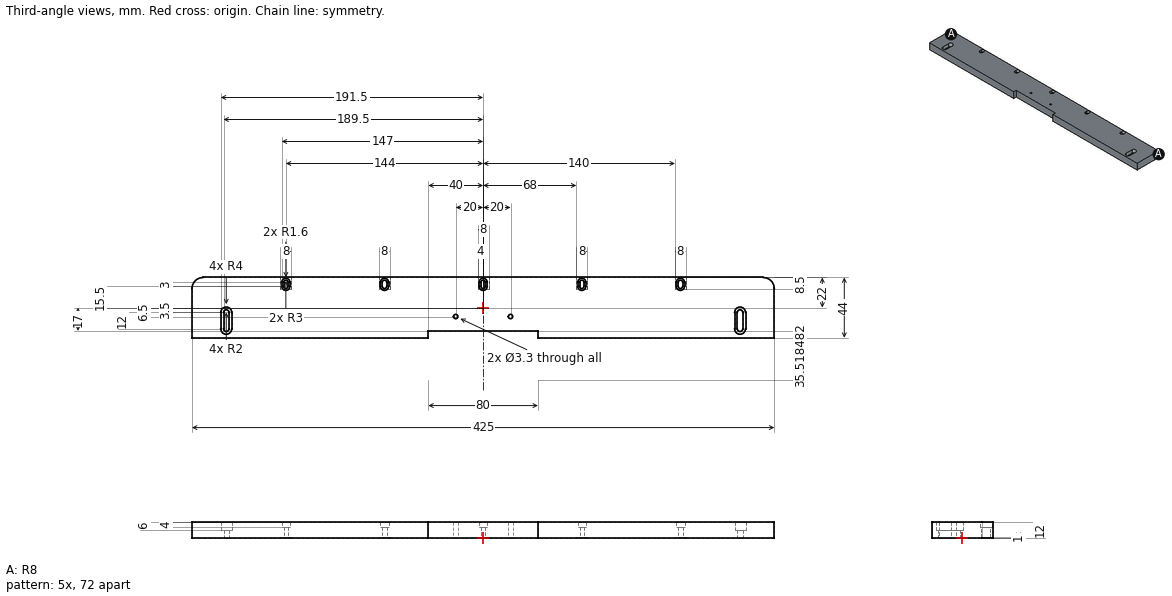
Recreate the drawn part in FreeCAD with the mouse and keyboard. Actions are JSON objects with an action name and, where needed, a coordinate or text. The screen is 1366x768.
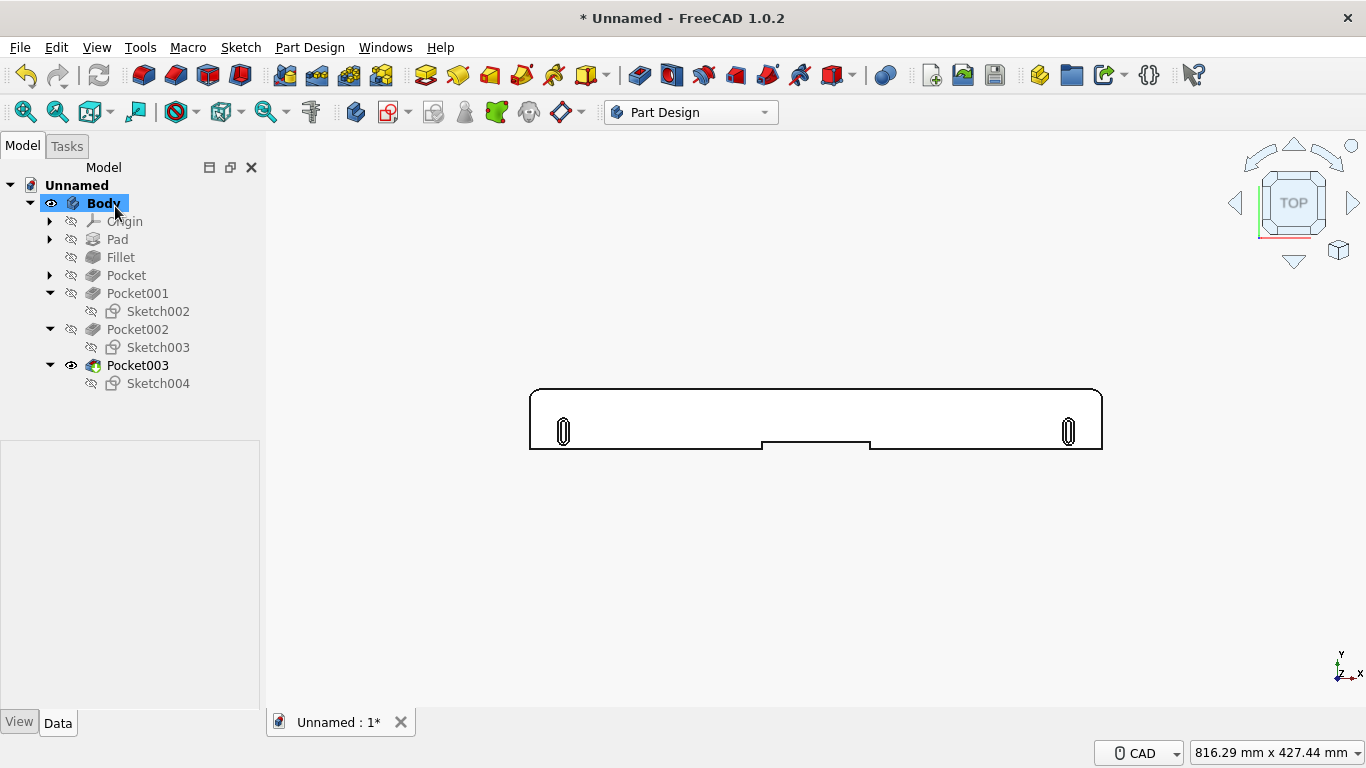
{"action": "left_click", "coordinate": [980, 418]}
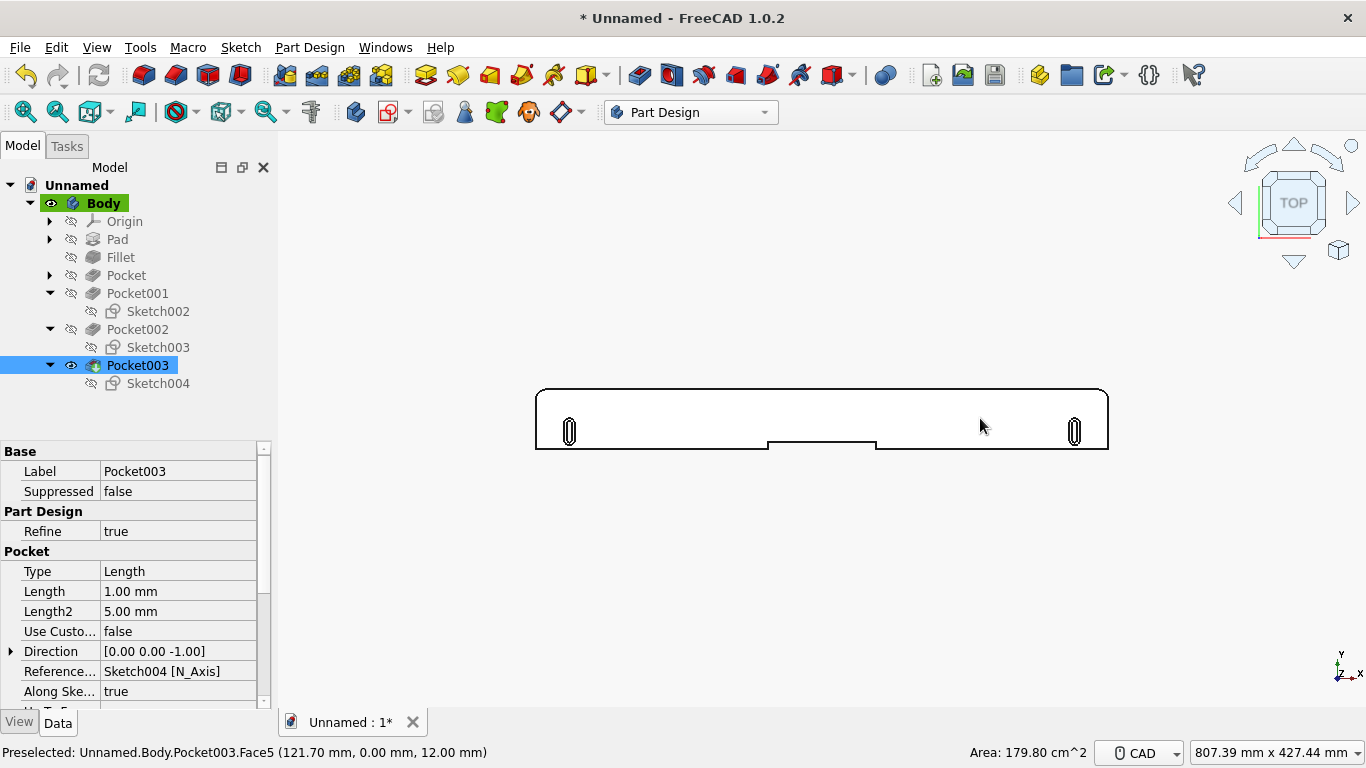
{"action": "left_click", "coordinate": [388, 112]}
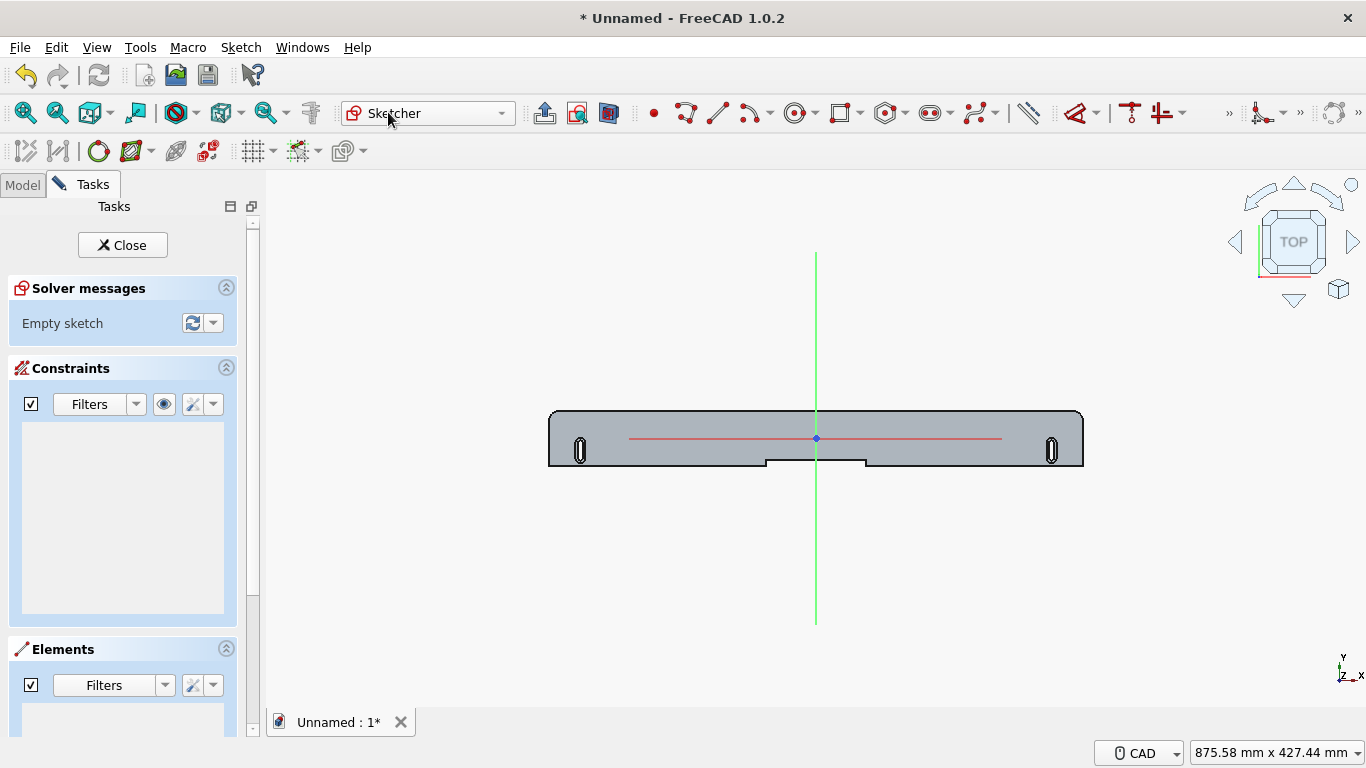
{"action": "scroll", "coordinate": [629, 416], "scroll_direction": "up", "scroll_amount": 15}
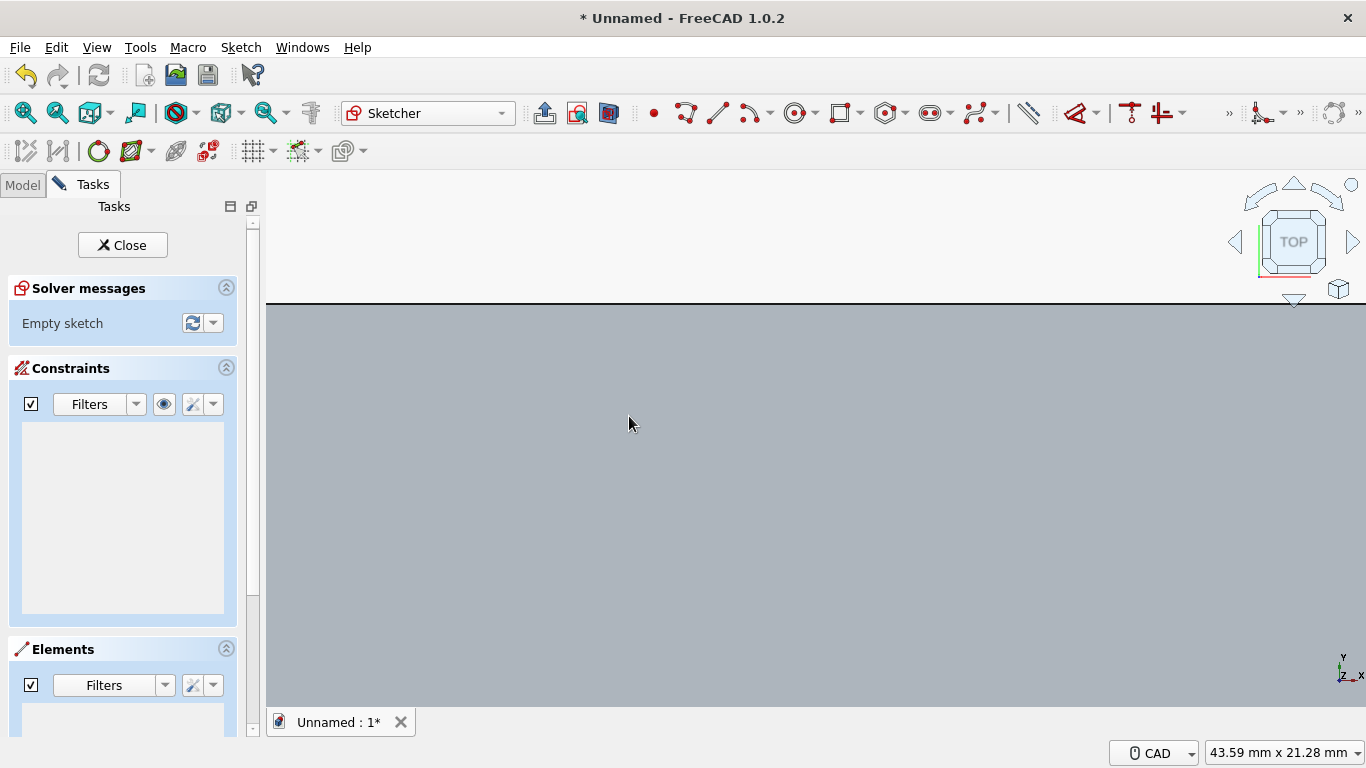
{"action": "scroll", "coordinate": [740, 413], "scroll_direction": "up", "scroll_amount": 2}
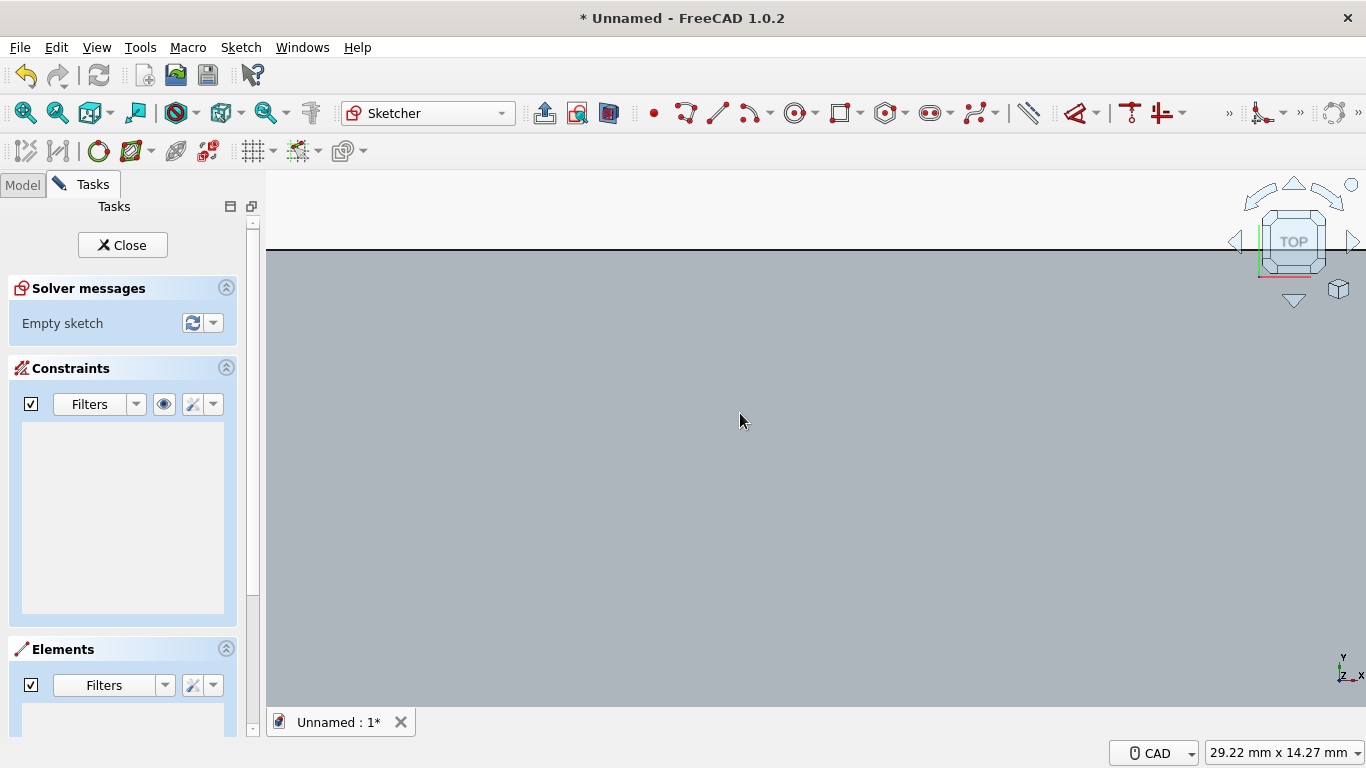
{"action": "left_click", "coordinate": [930, 114]}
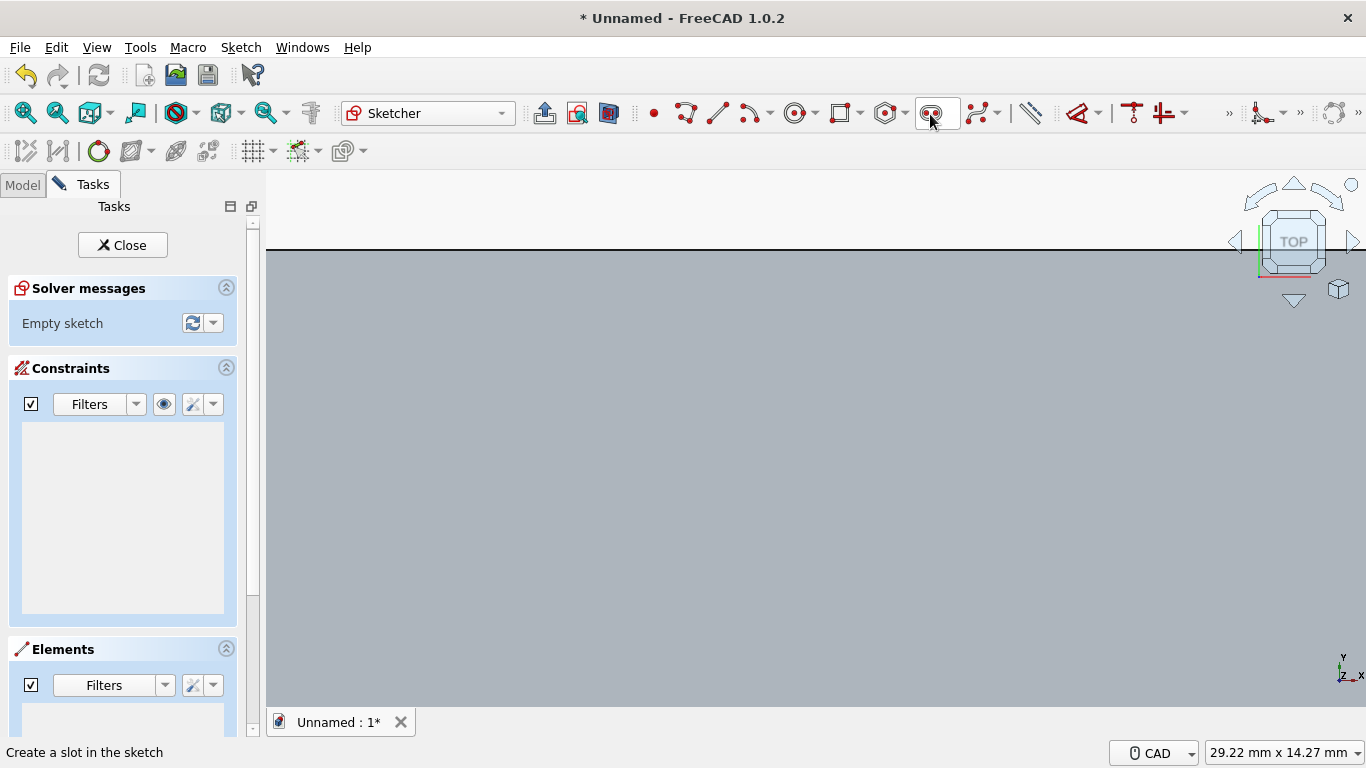
{"action": "left_click", "coordinate": [747, 495]}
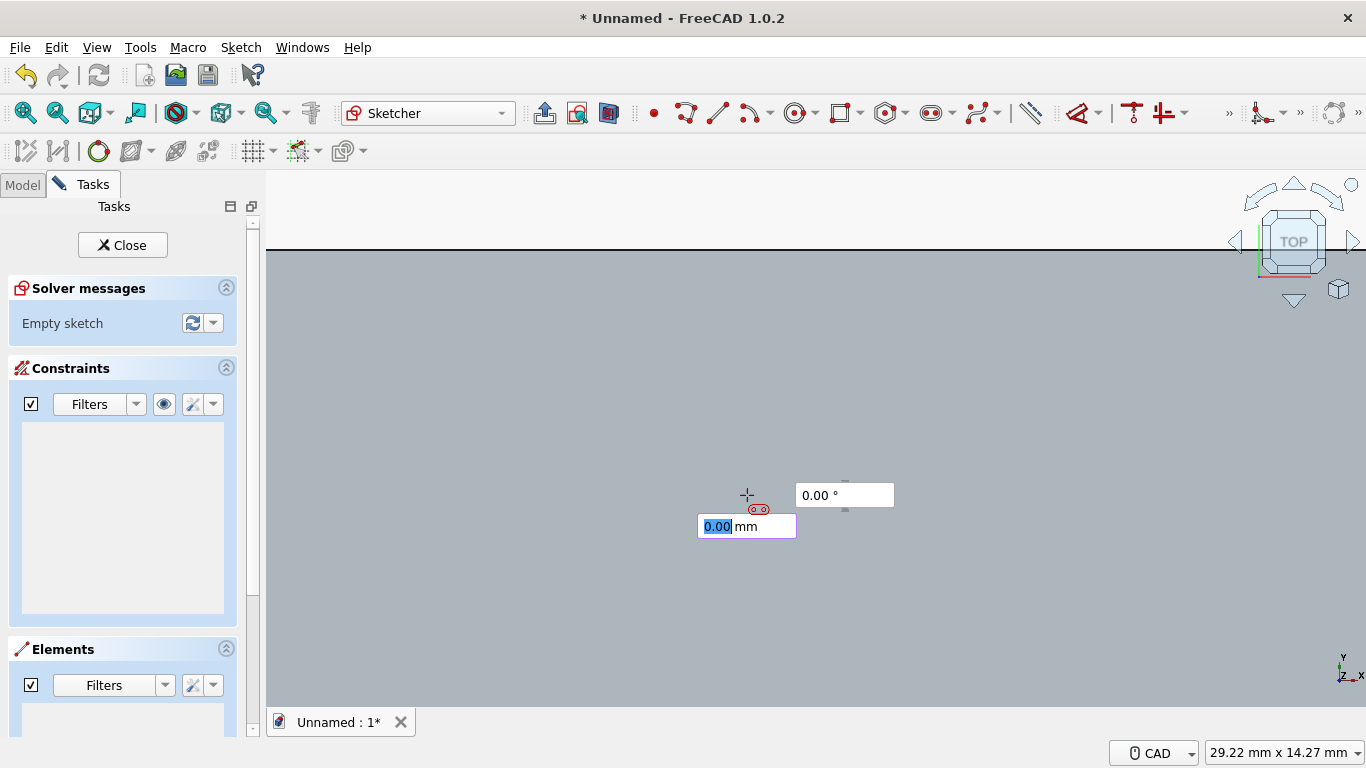
{"action": "left_click", "coordinate": [747, 382]}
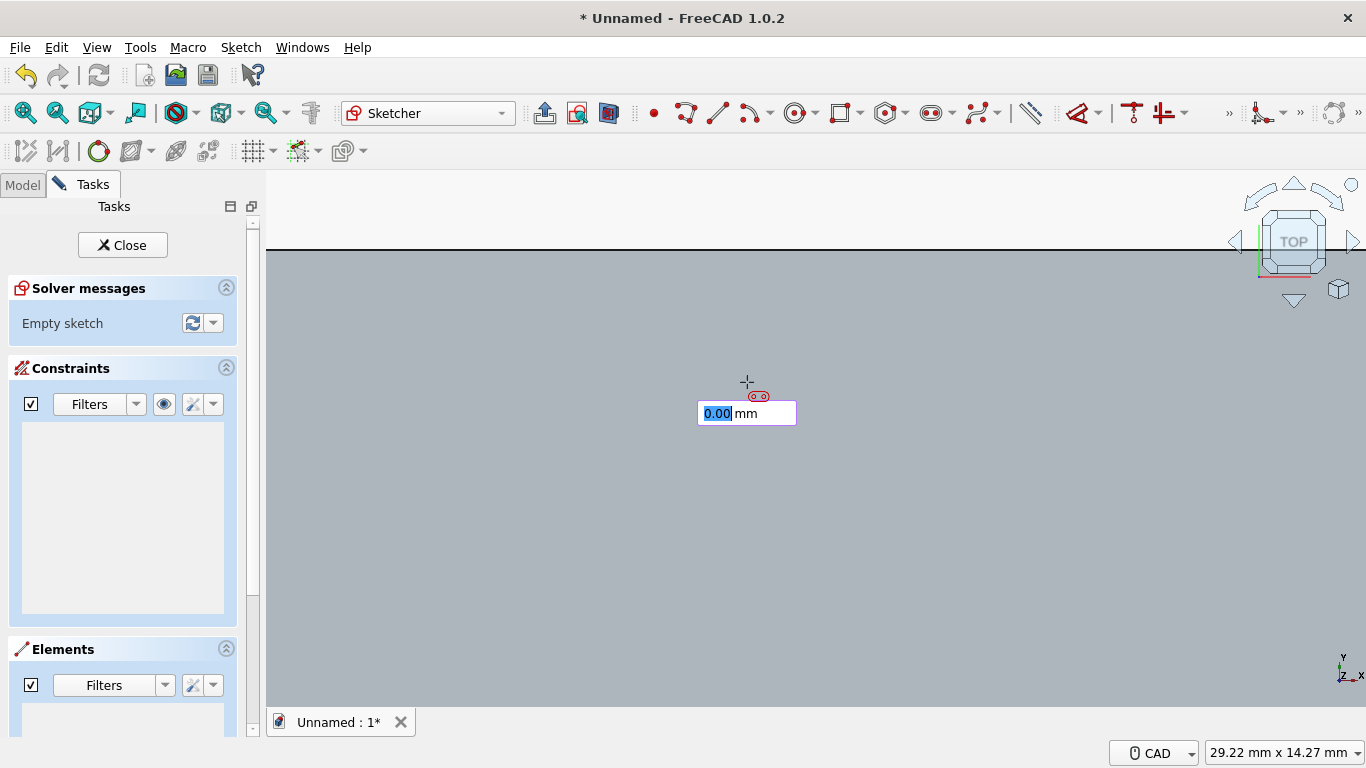
{"action": "left_click", "coordinate": [860, 438]}
{"action": "key", "text": "Escape"}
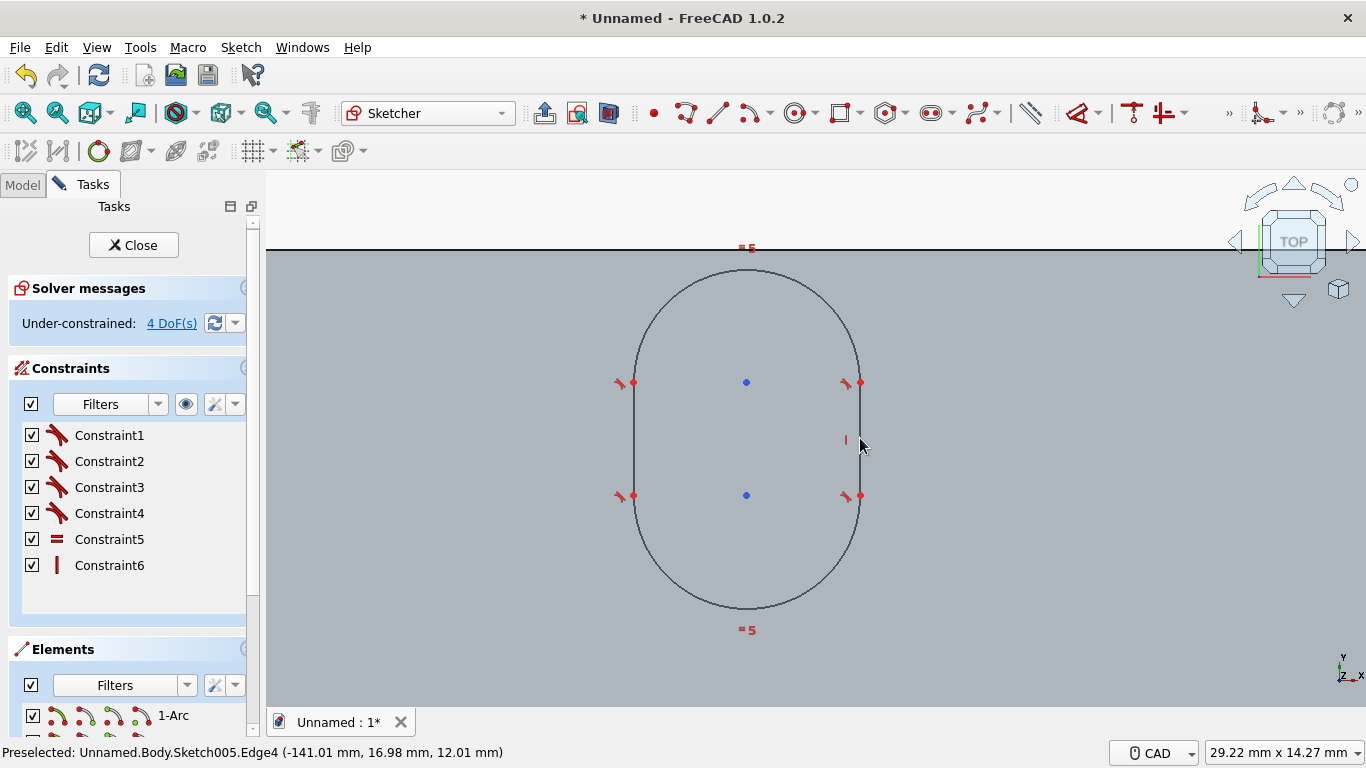
{"action": "key", "text": "d"}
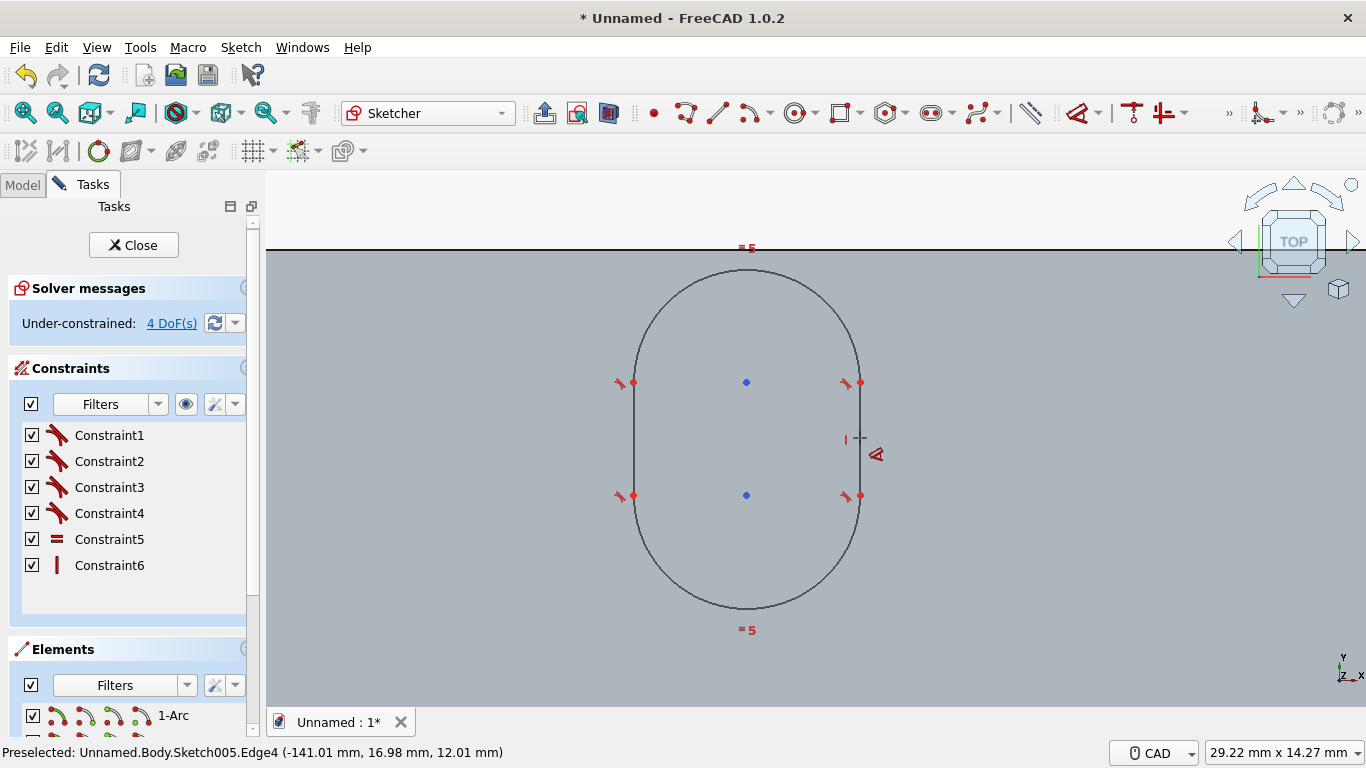
{"action": "left_click", "coordinate": [681, 587]}
{"action": "left_click", "coordinate": [662, 613]}